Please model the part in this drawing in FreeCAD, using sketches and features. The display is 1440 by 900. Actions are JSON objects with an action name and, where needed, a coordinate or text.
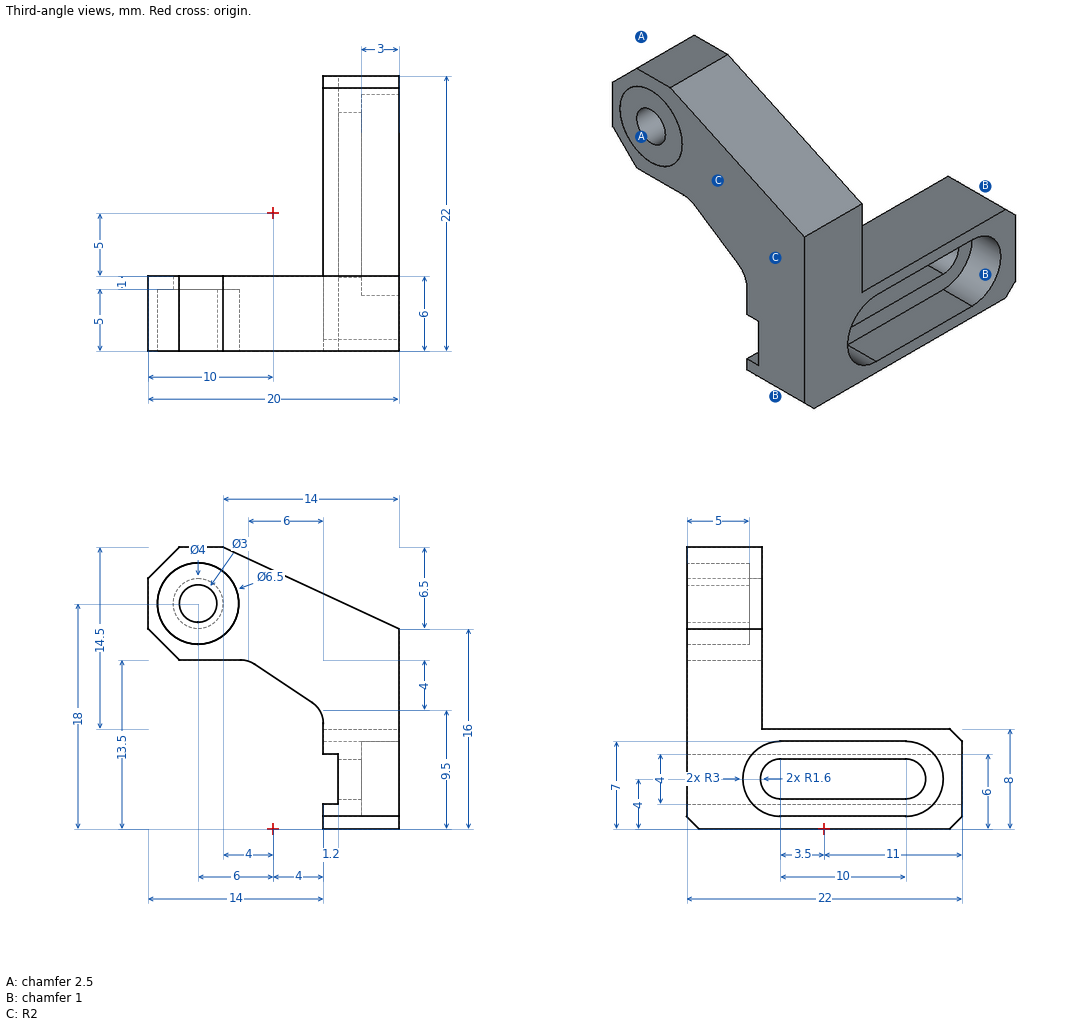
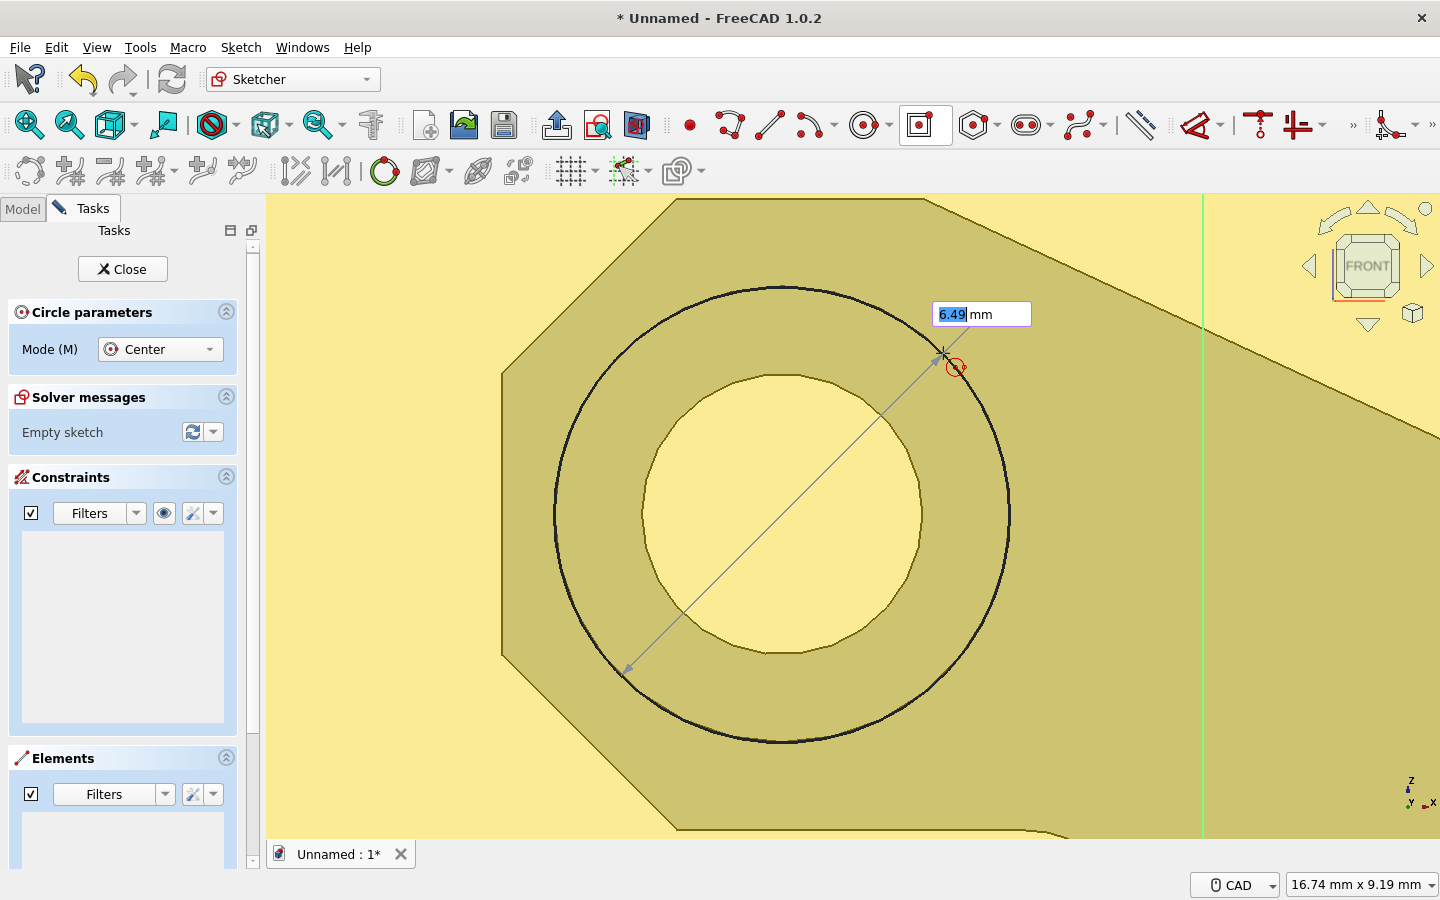
{"action": "type", "text": "6.5"}
{"action": "key", "text": "Return"}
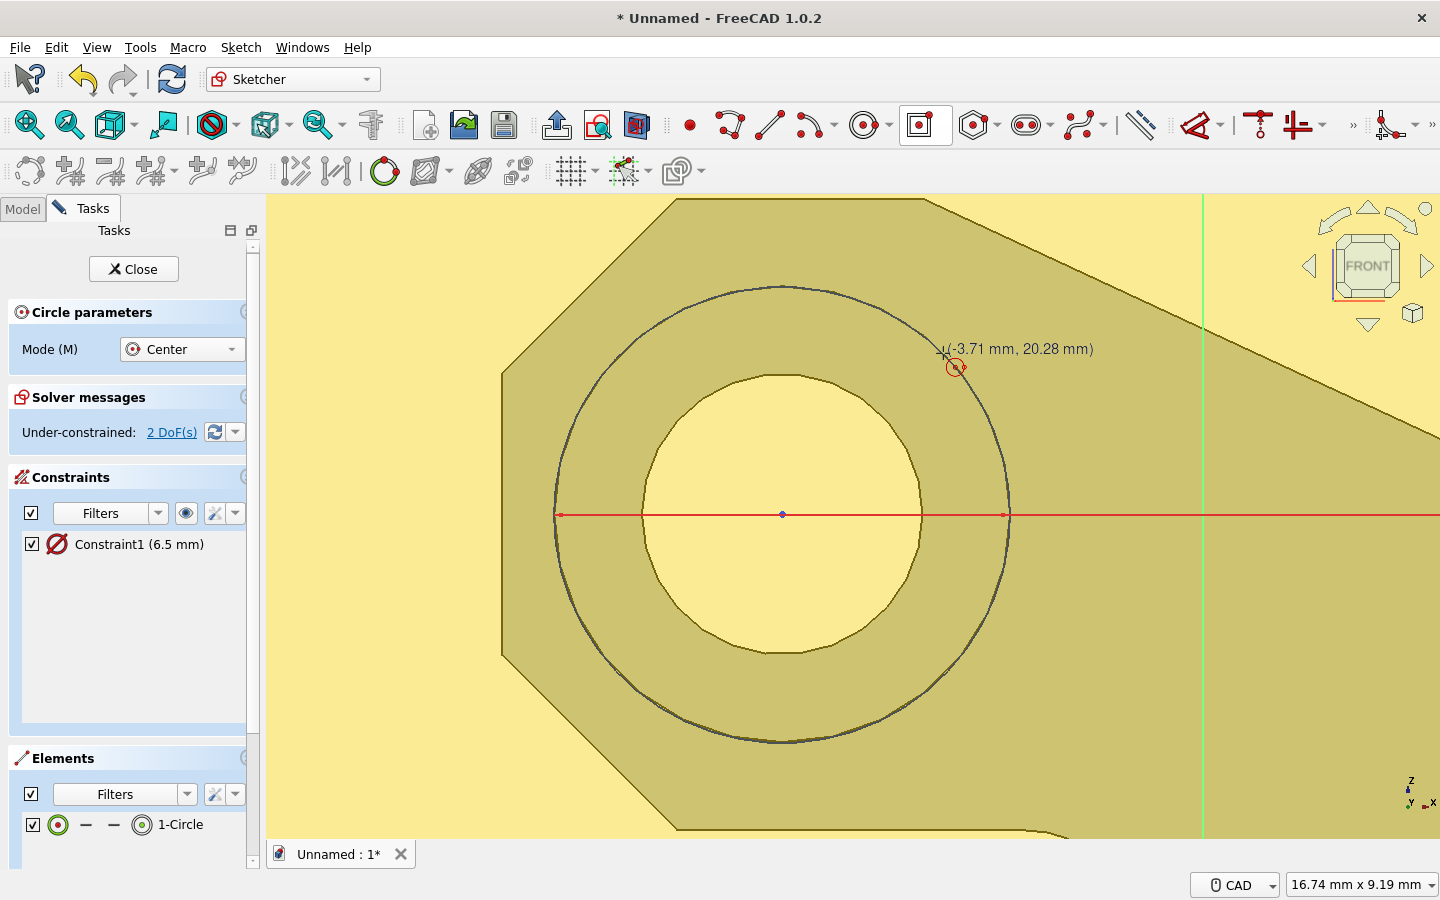
{"action": "left_click", "coordinate": [782, 515]}
{"action": "mouse_move", "coordinate": [857, 440]}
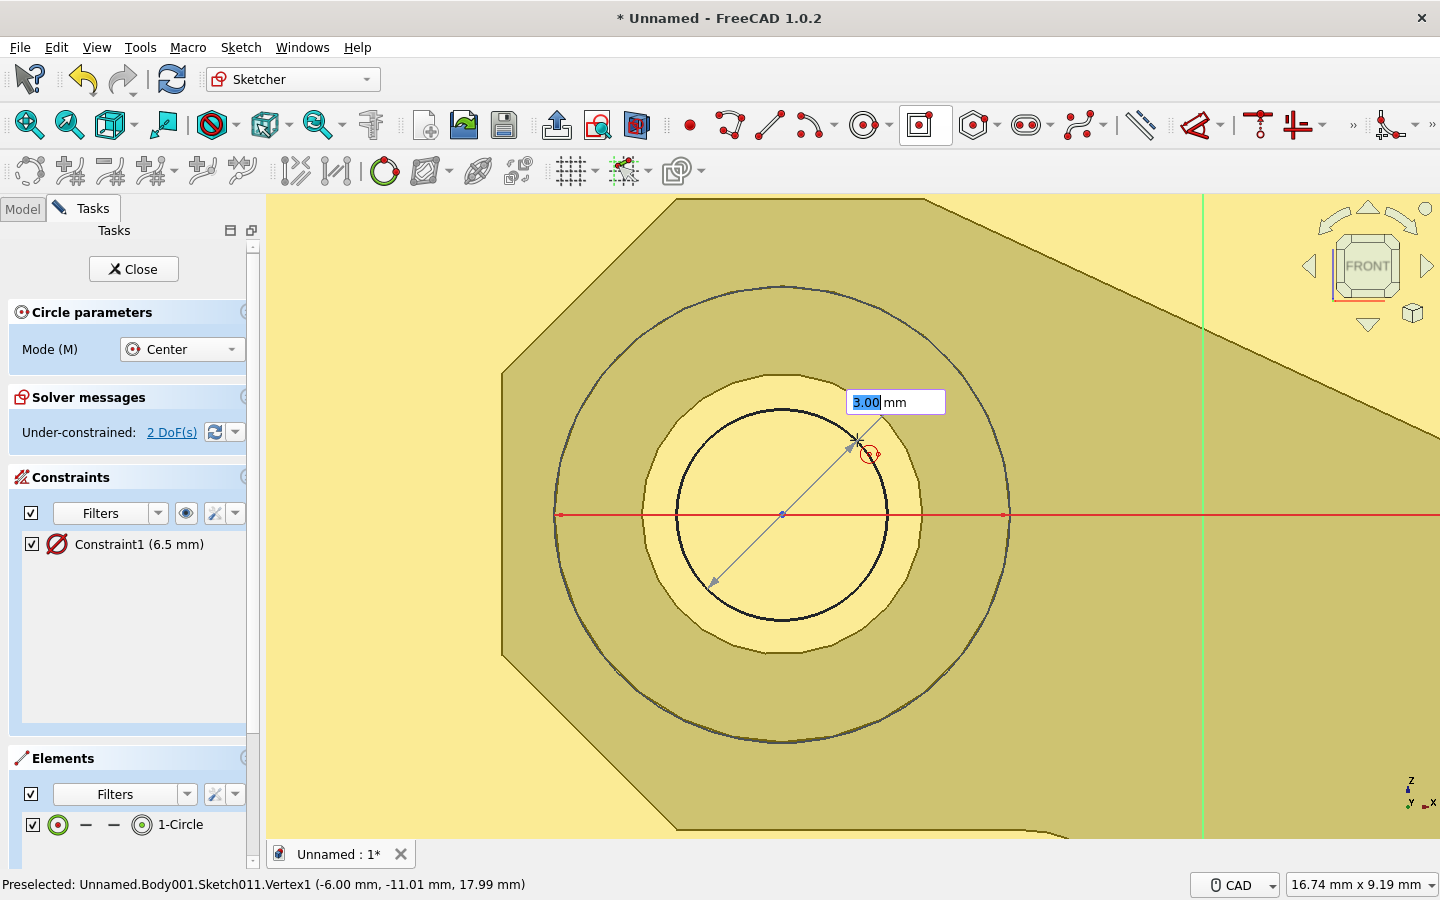
{"action": "type", "text": "3"}
{"action": "key", "text": "Return"}
{"action": "key", "text": "Escape"}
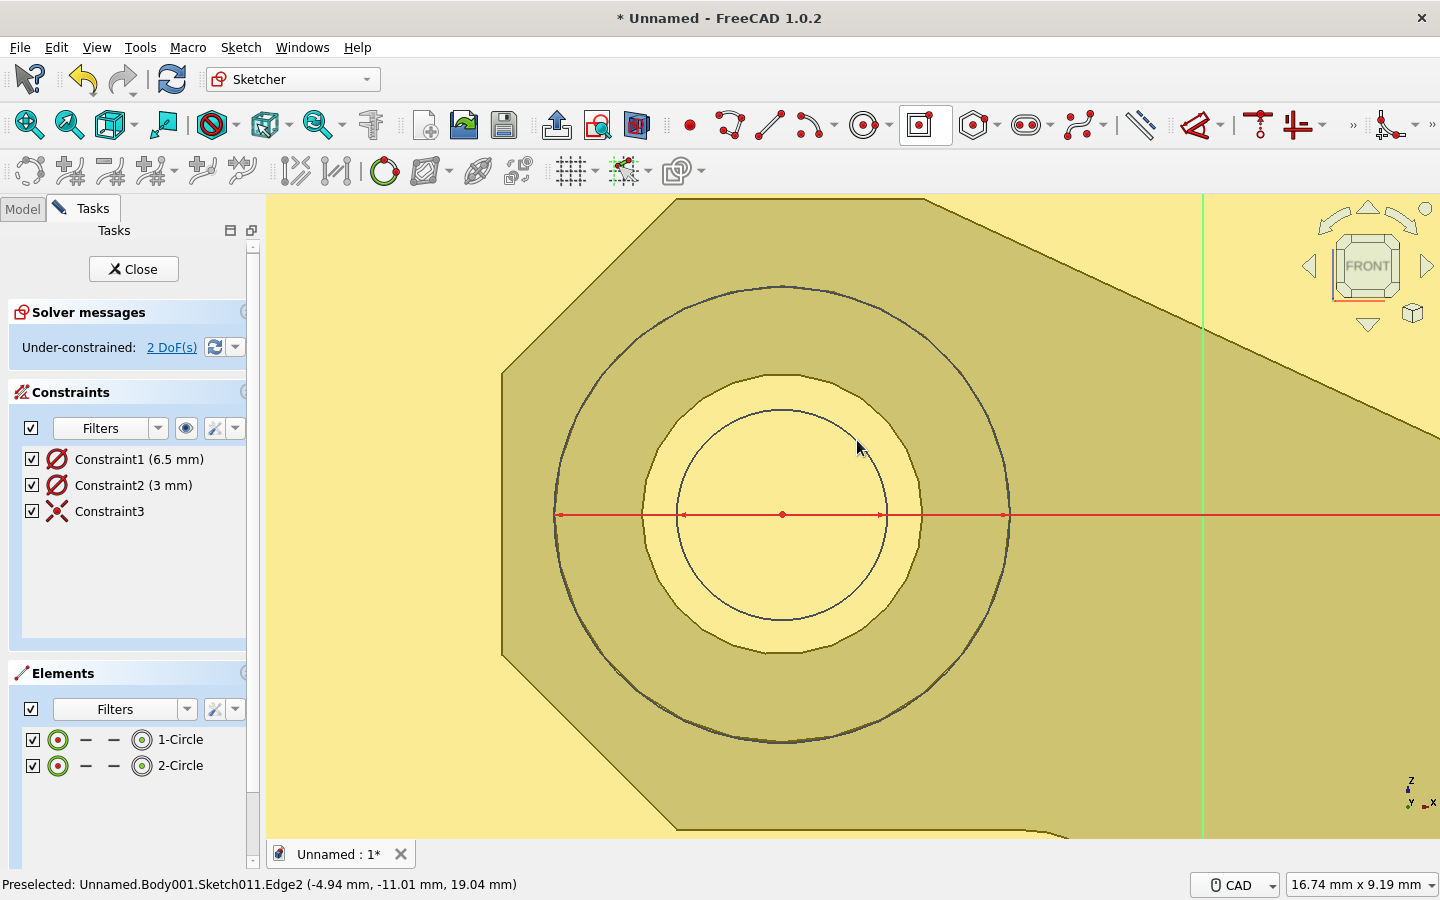
{"action": "left_click", "coordinate": [1196, 126]}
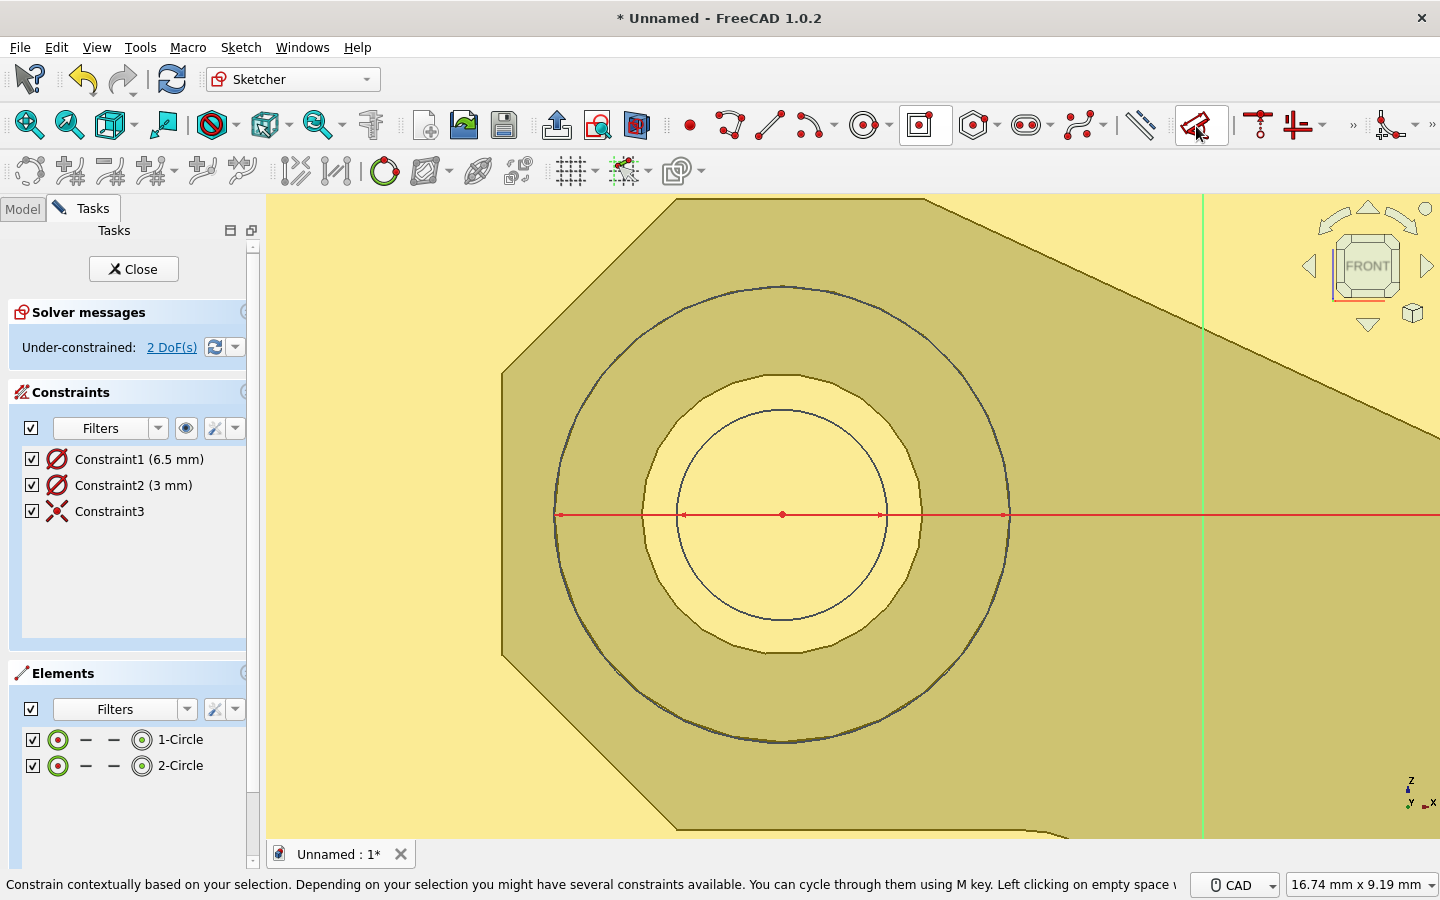
{"action": "left_click", "coordinate": [782, 515]}
{"action": "left_click", "coordinate": [993, 481]}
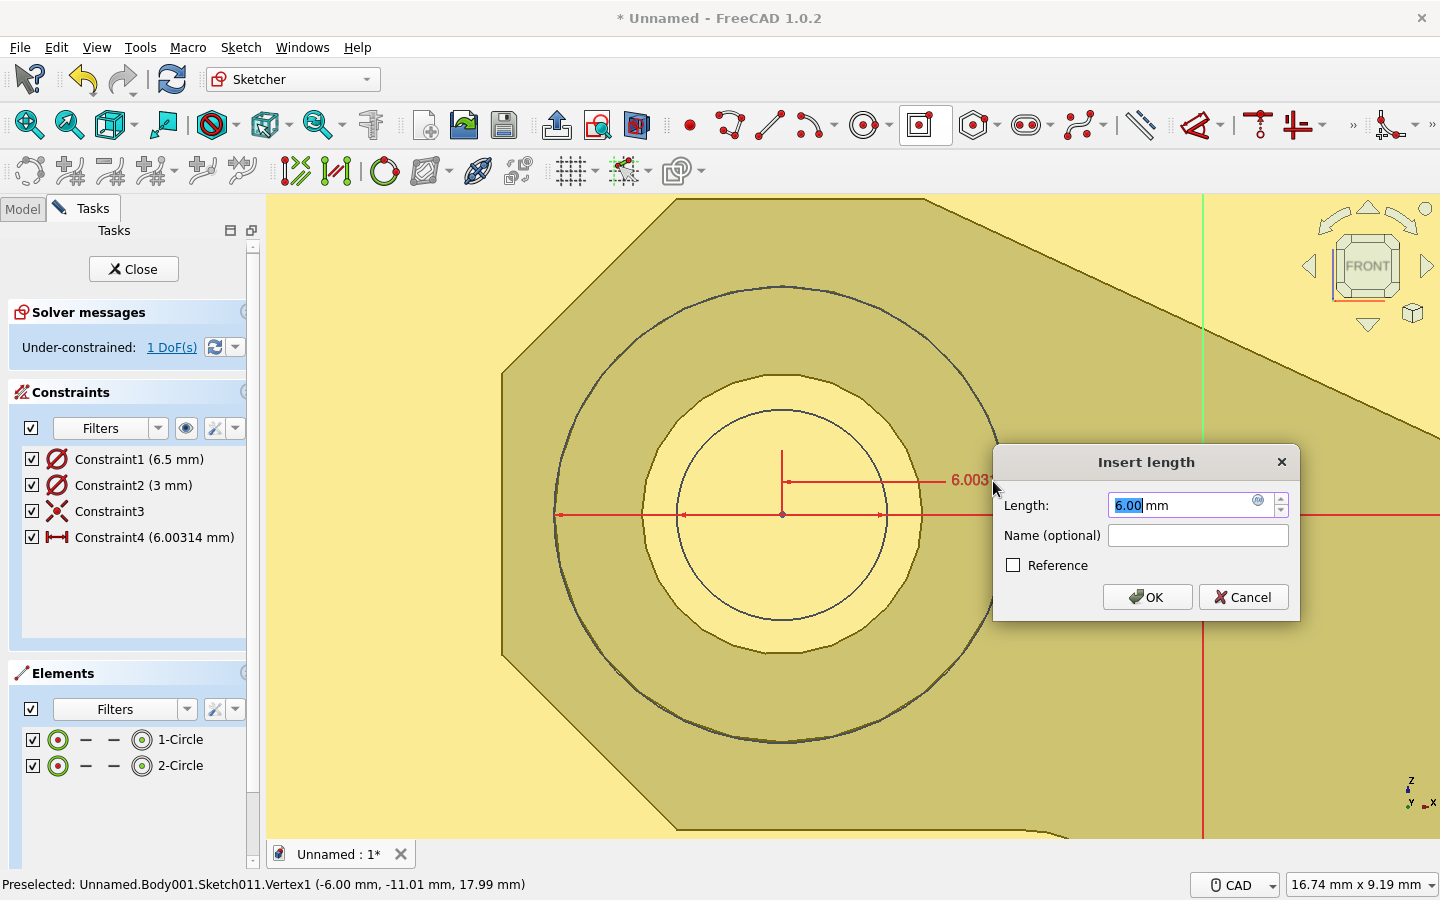
{"action": "type", "text": "6"}
{"action": "key", "text": "Return"}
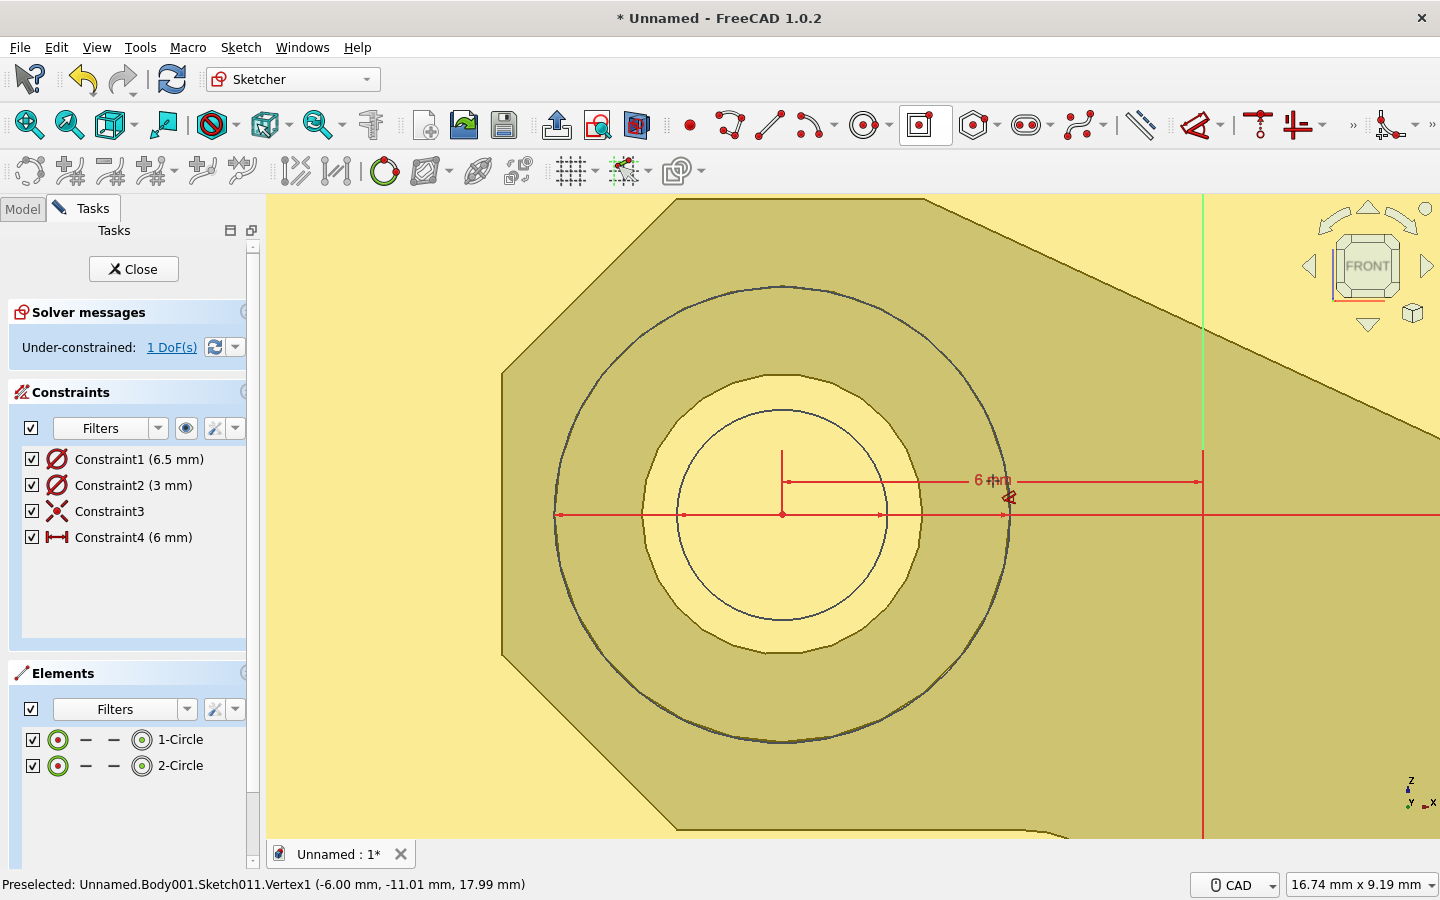
{"action": "left_click", "coordinate": [782, 515]}
{"action": "left_click", "coordinate": [1237, 663]}